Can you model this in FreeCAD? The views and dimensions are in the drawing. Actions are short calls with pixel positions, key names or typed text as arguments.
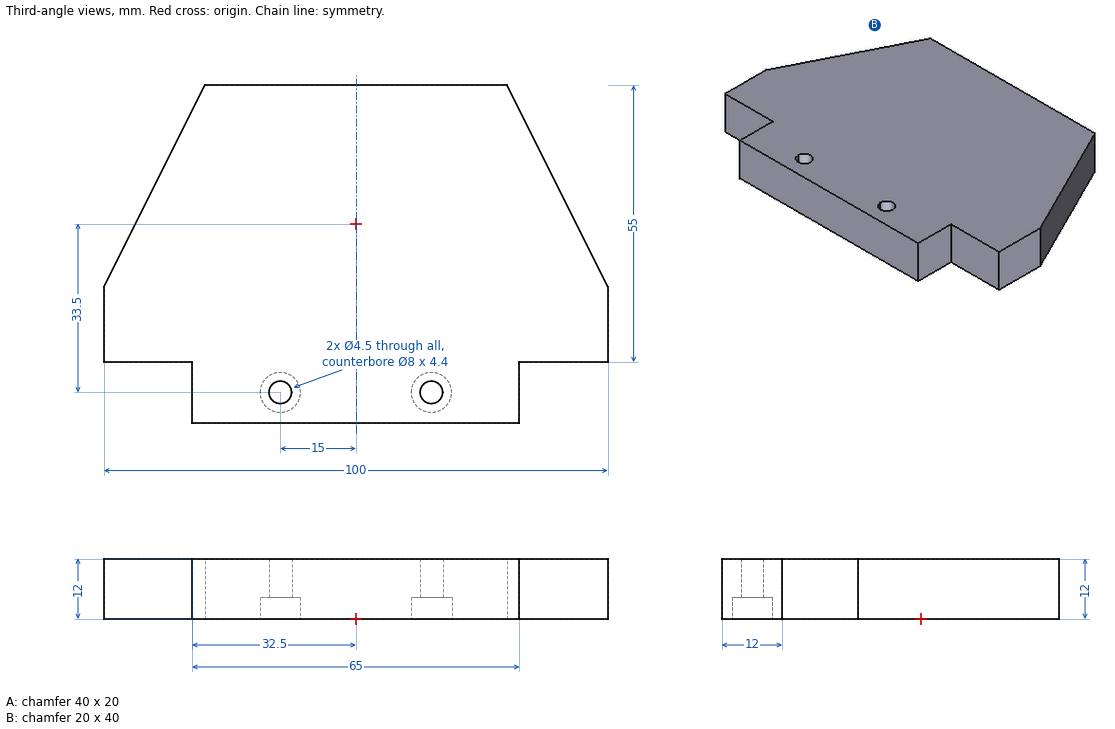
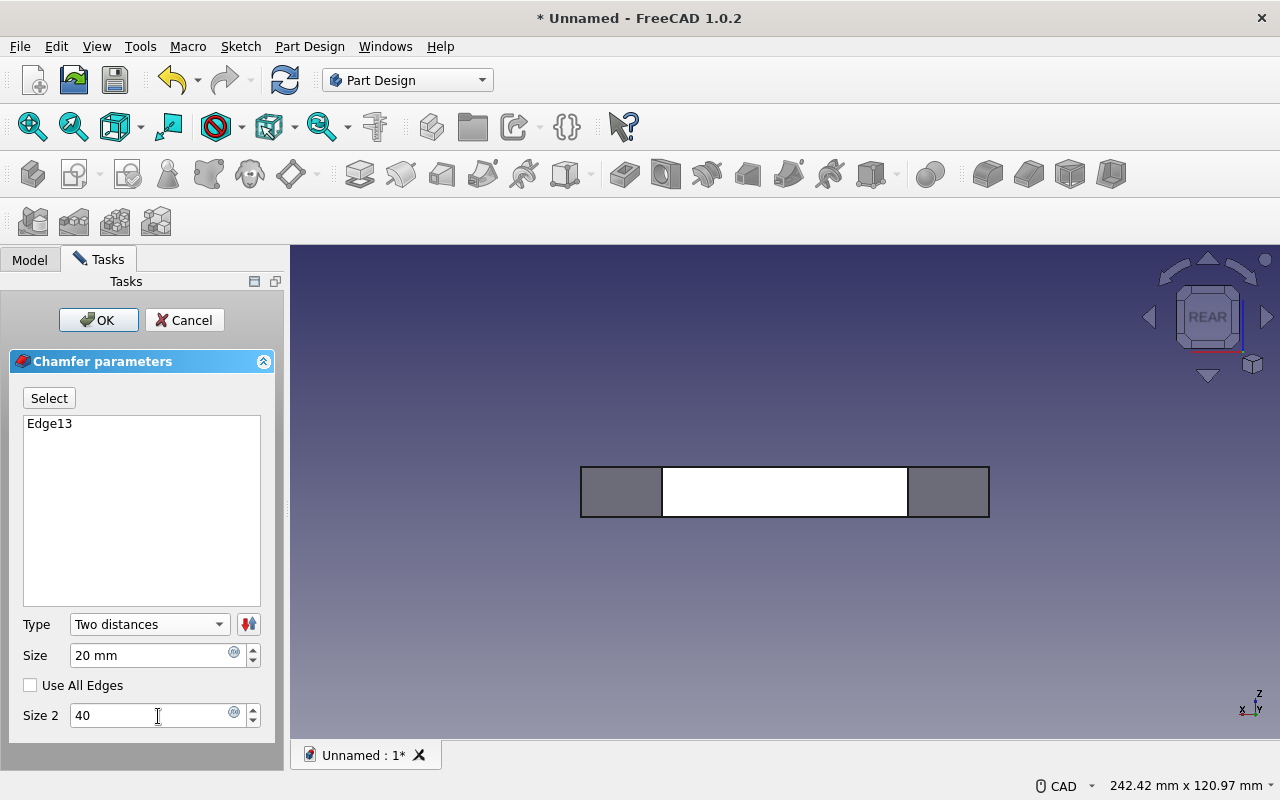
click(99, 320)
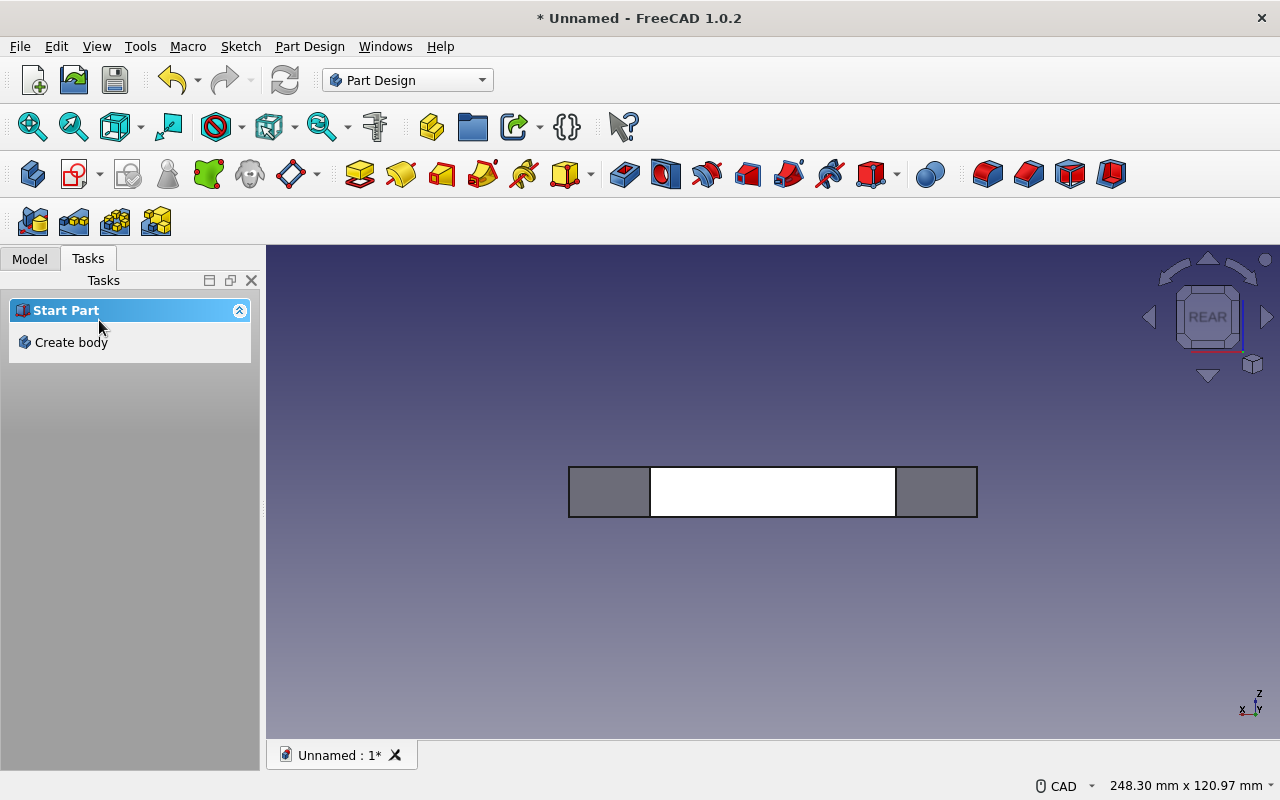
key(0)